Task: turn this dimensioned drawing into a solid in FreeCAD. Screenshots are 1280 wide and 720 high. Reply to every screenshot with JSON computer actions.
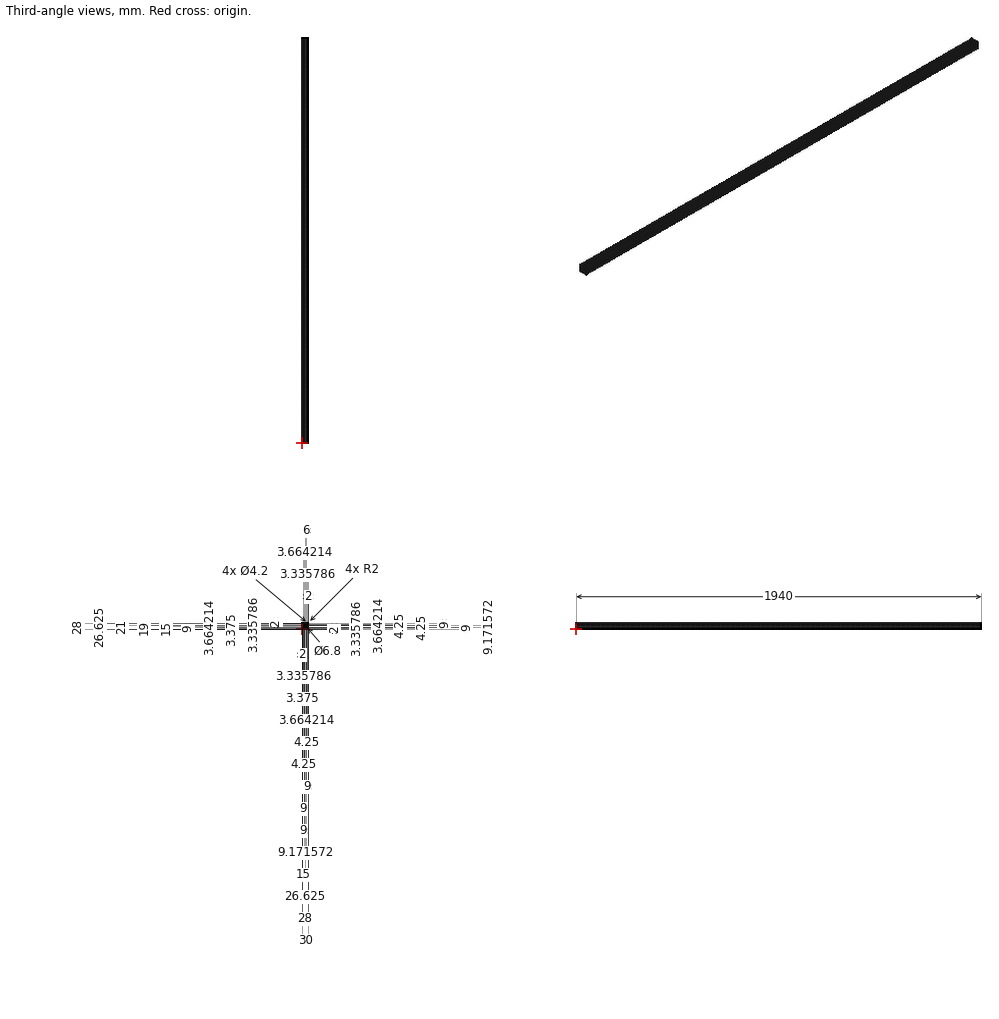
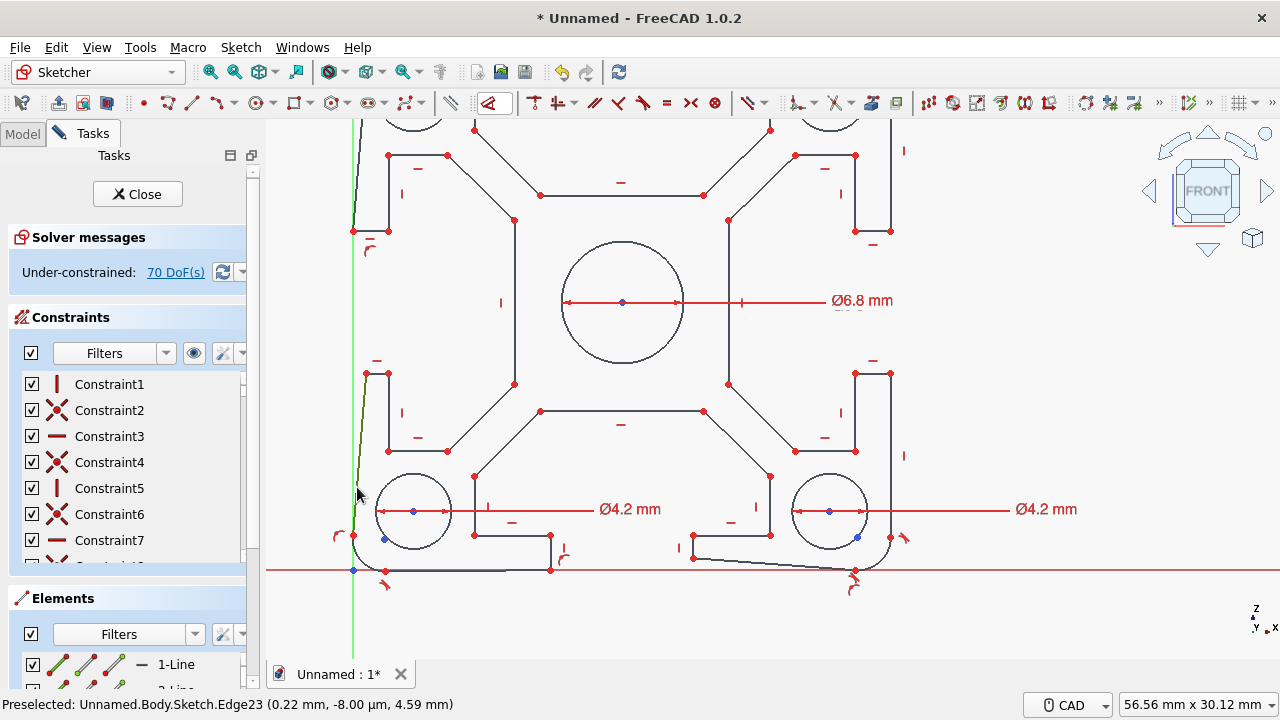
{"action": "left_click", "coordinate": [355, 551]}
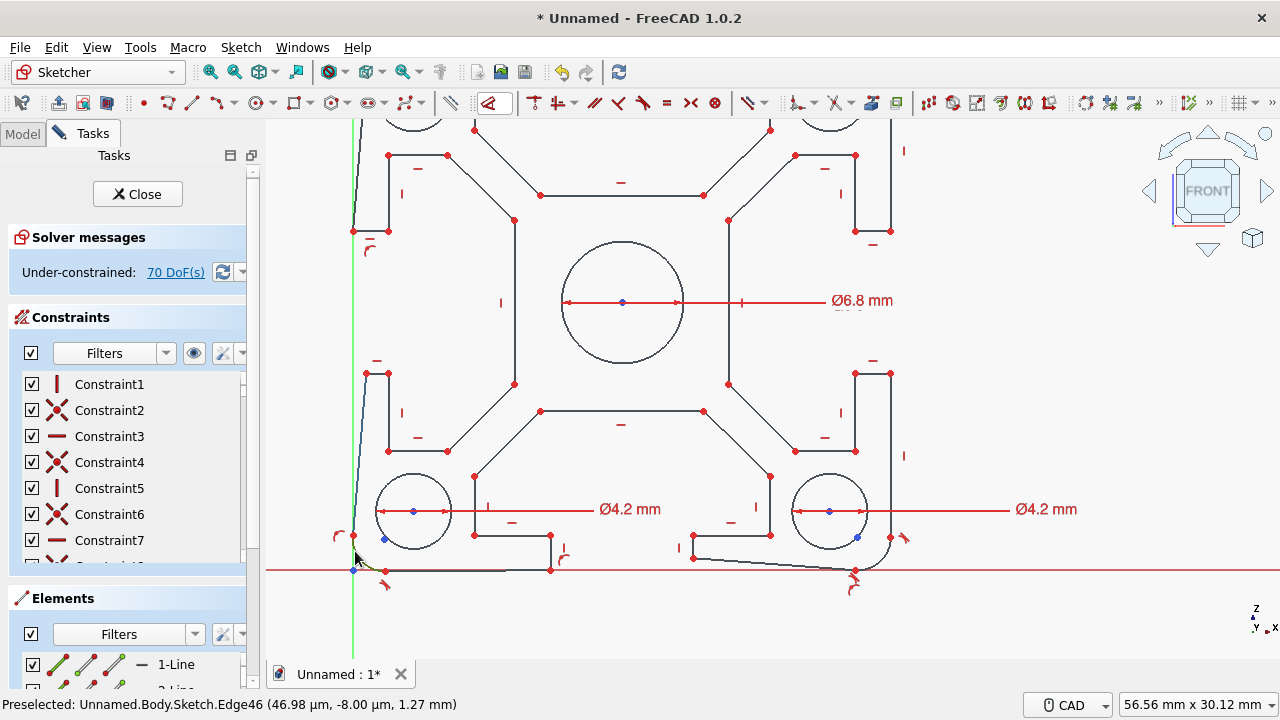
{"action": "left_click", "coordinate": [644, 104]}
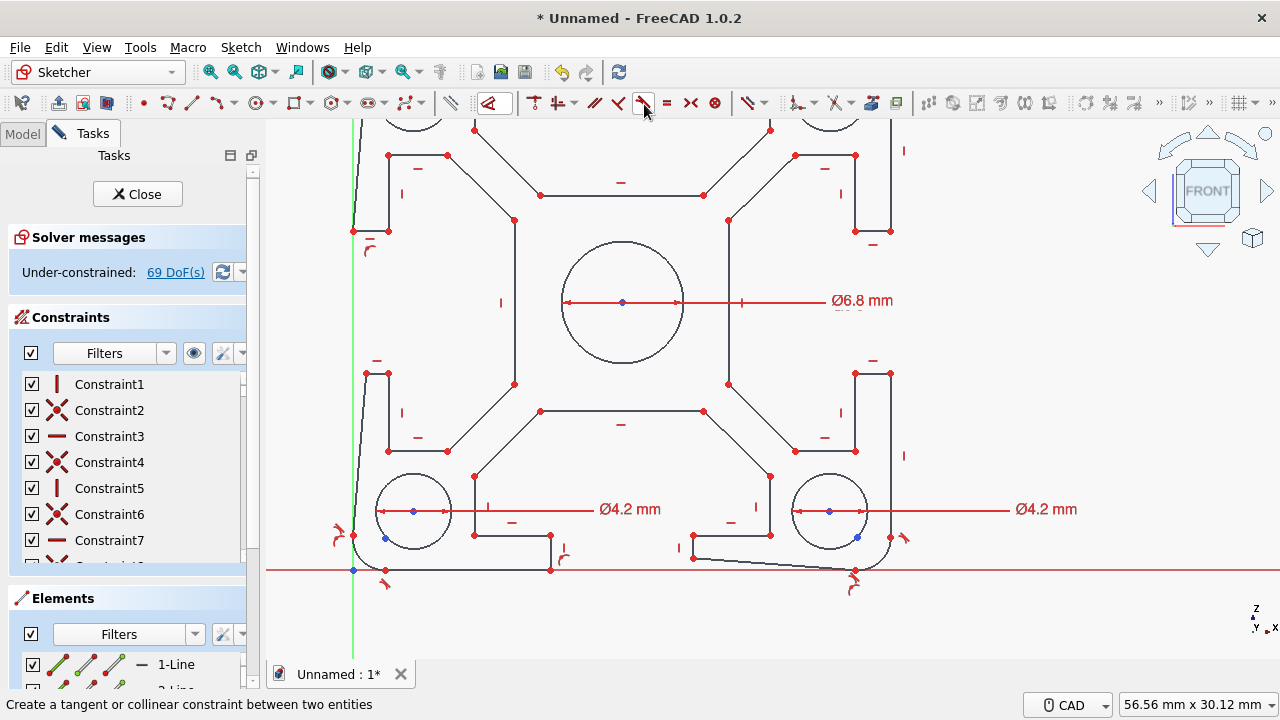
{"action": "left_click", "coordinate": [357, 183]}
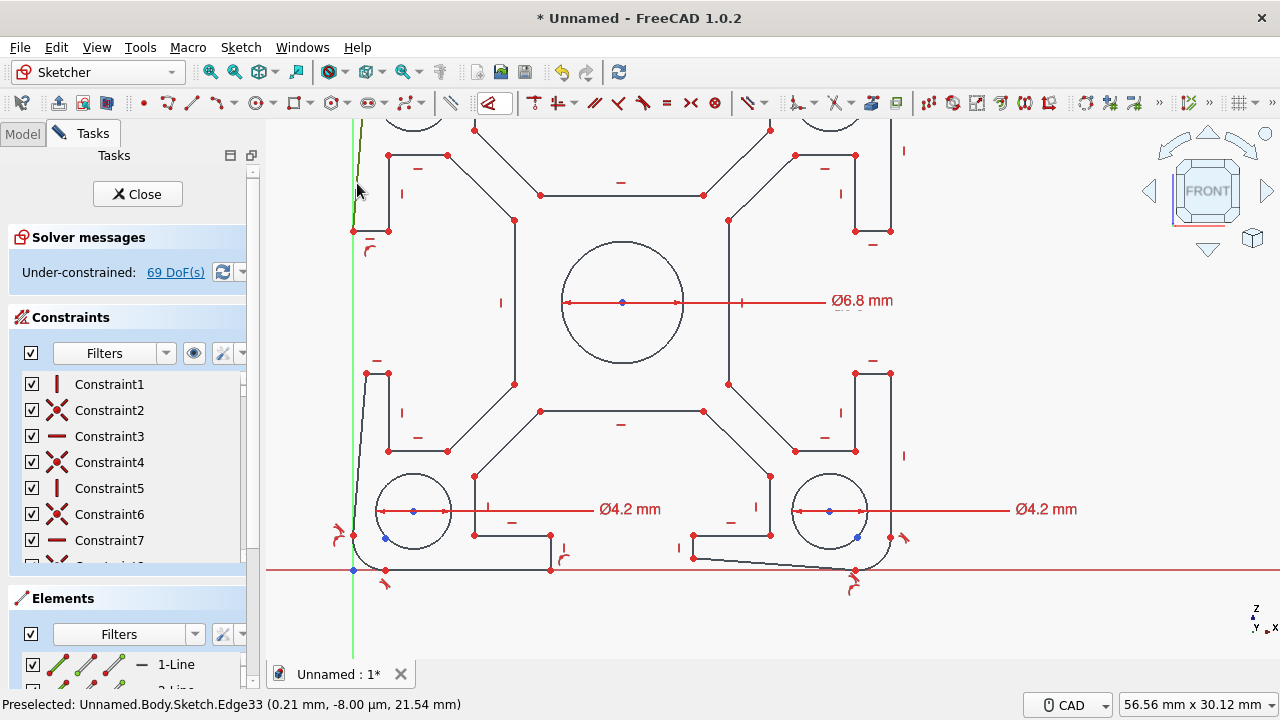
{"action": "scroll", "coordinate": [872, 567], "scroll_direction": "down", "scroll_amount": 2}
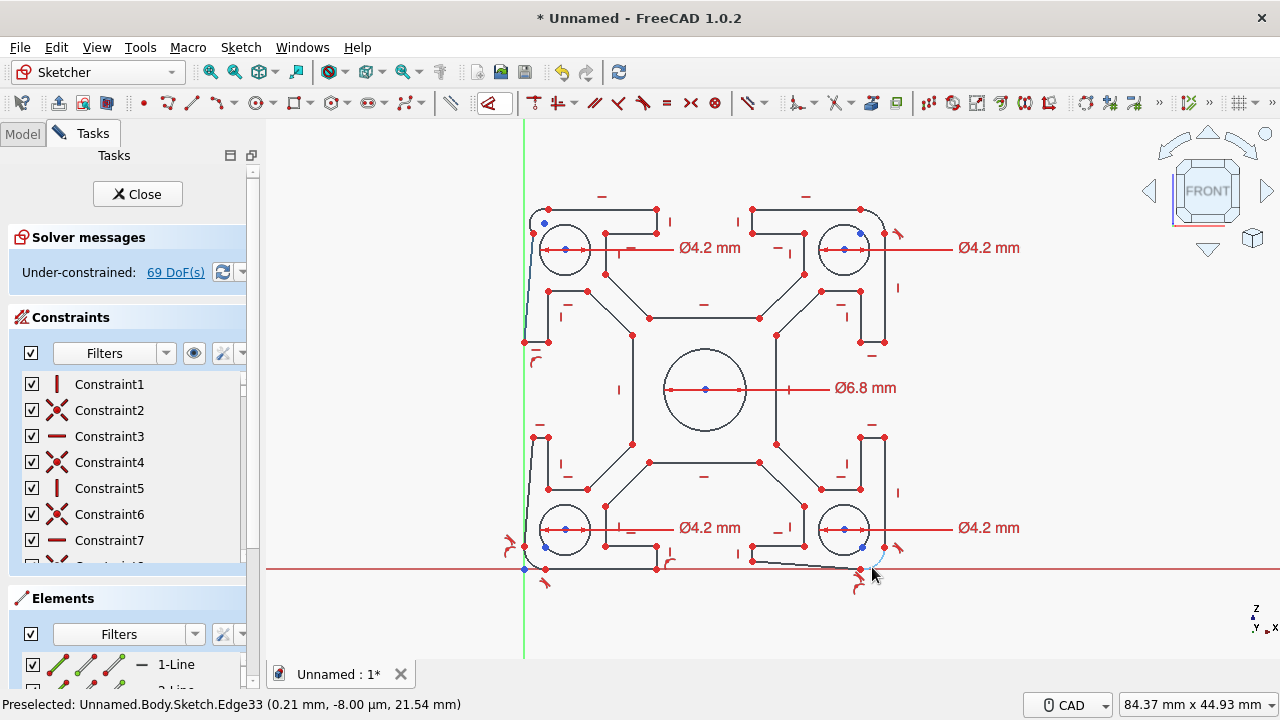
{"action": "scroll", "coordinate": [537, 211], "scroll_direction": "up", "scroll_amount": 2}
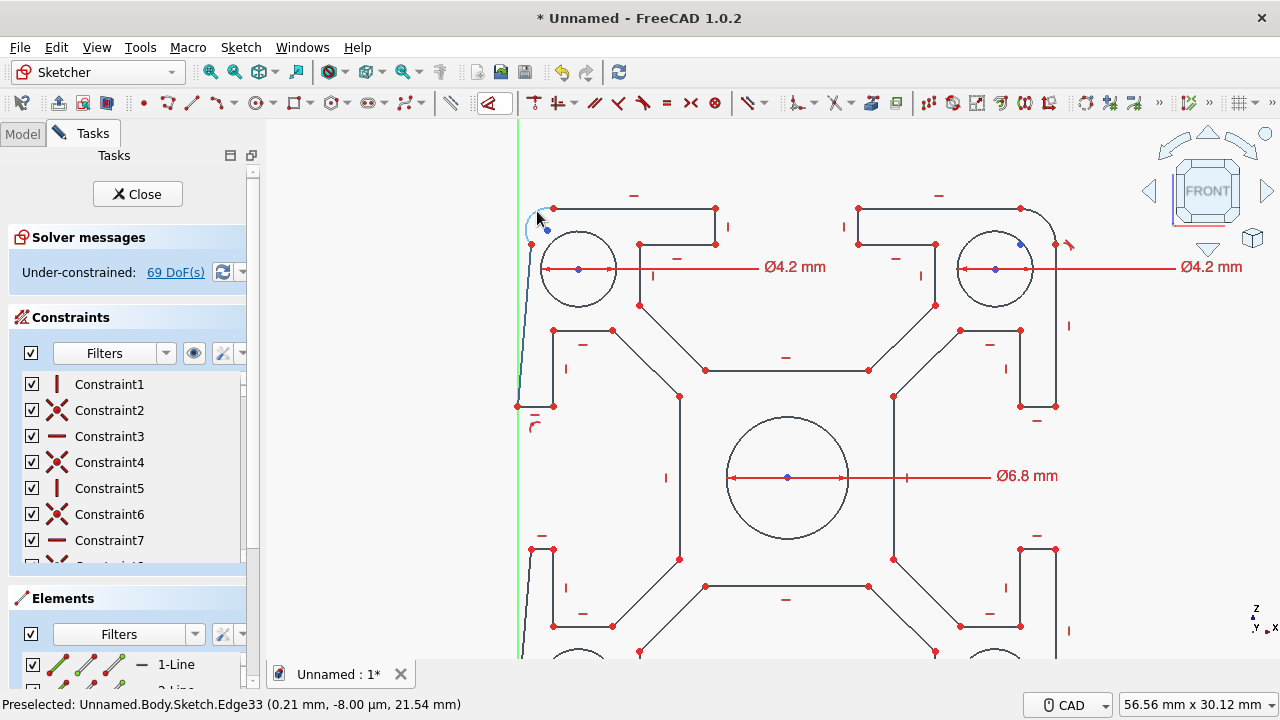
{"action": "left_click", "coordinate": [537, 211]}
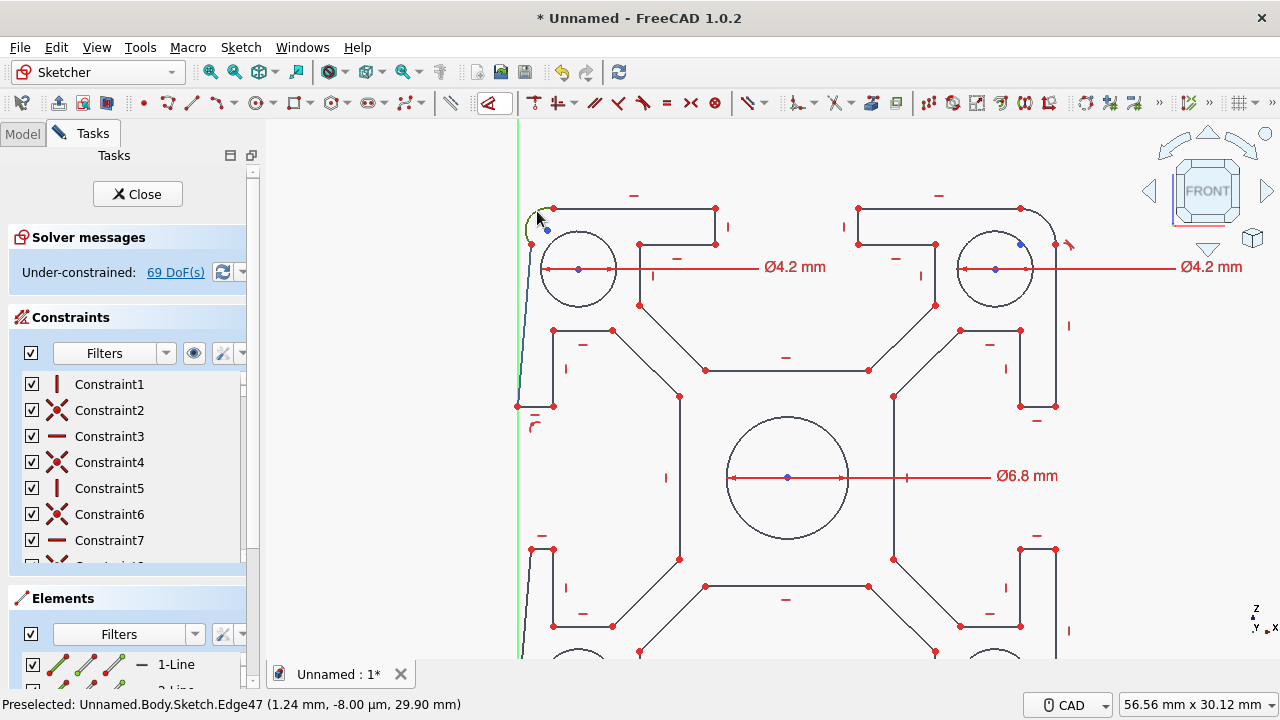
{"action": "left_click", "coordinate": [644, 104]}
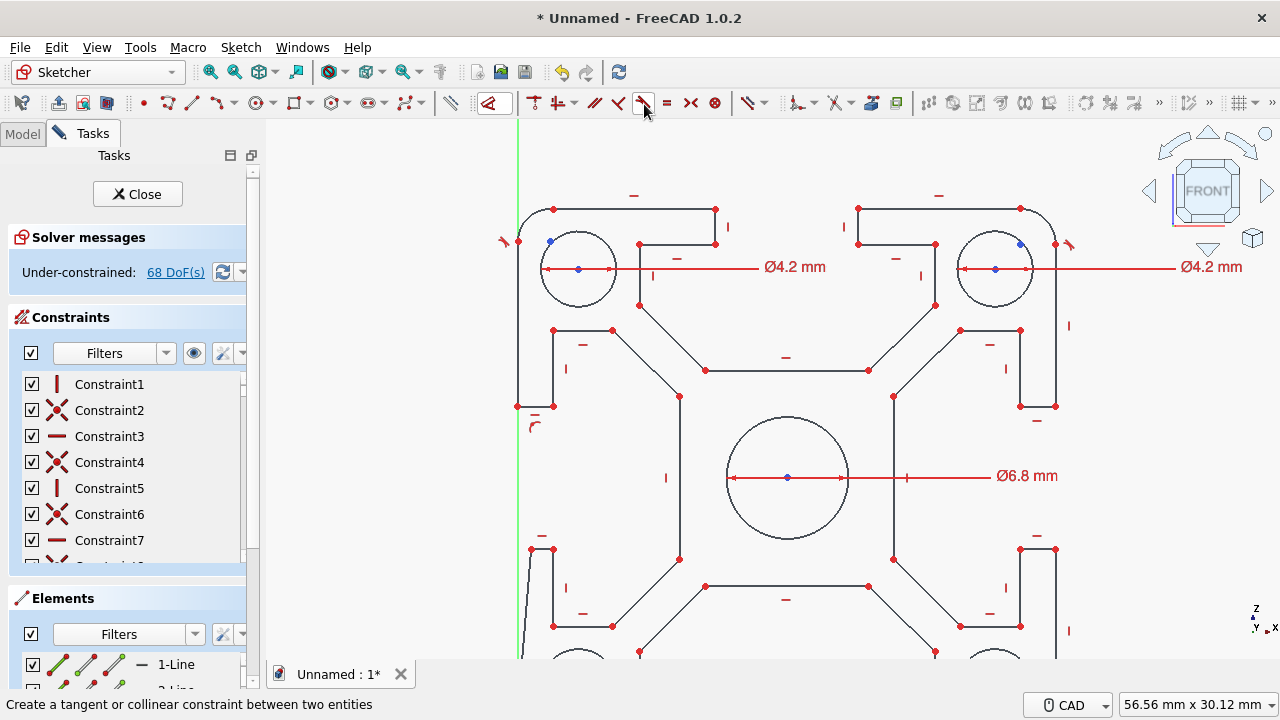
{"action": "left_click", "coordinate": [602, 209]}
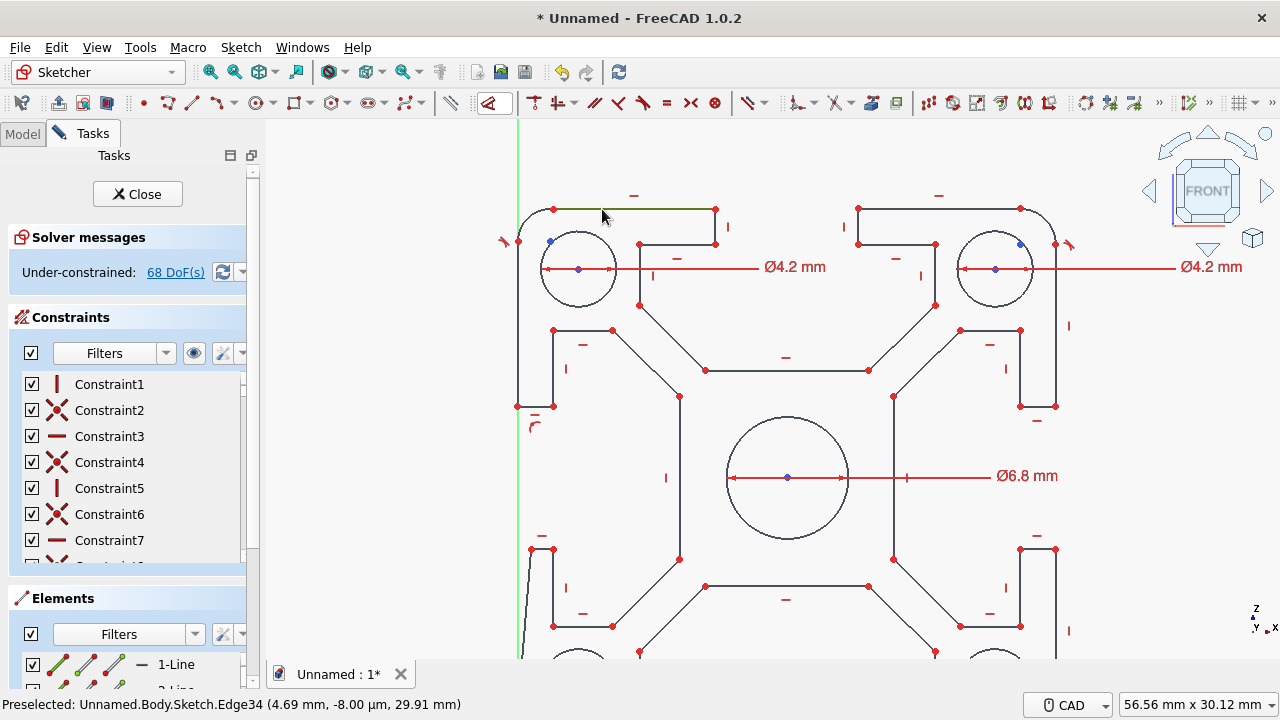
{"action": "left_click", "coordinate": [538, 212]}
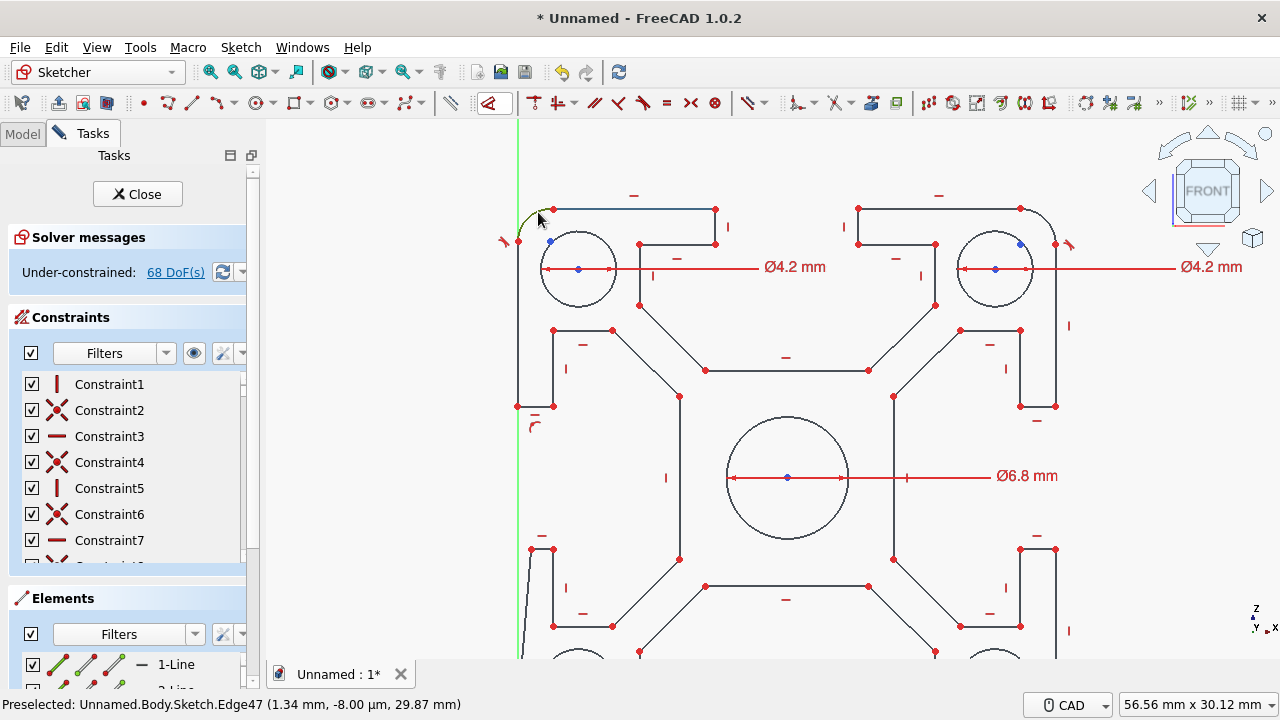
{"action": "left_click", "coordinate": [644, 104]}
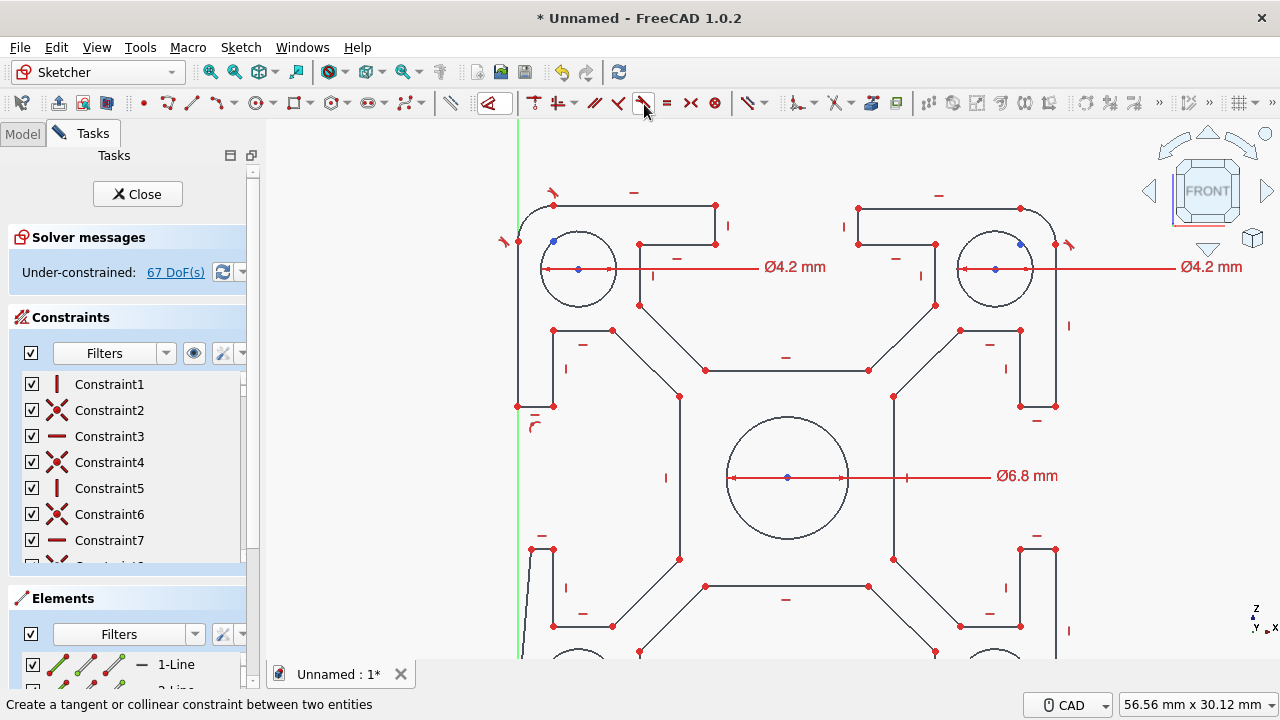
{"action": "left_click", "coordinate": [907, 209]}